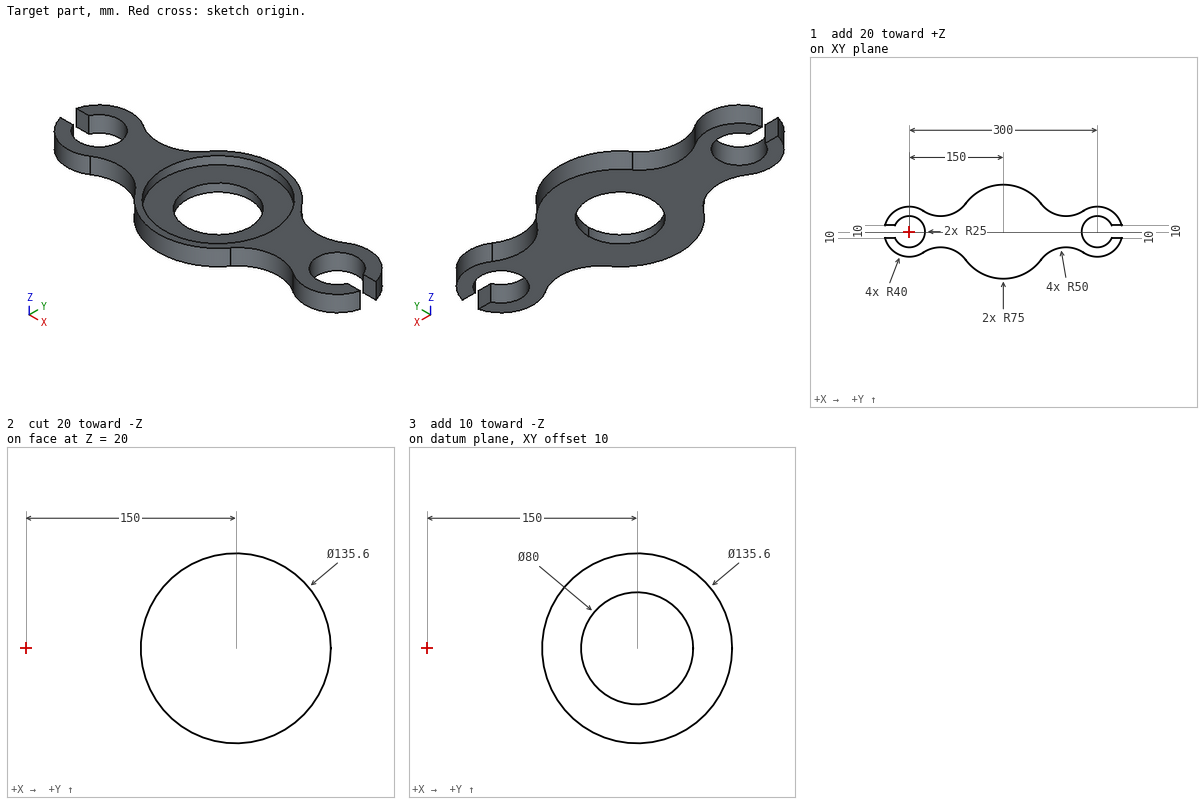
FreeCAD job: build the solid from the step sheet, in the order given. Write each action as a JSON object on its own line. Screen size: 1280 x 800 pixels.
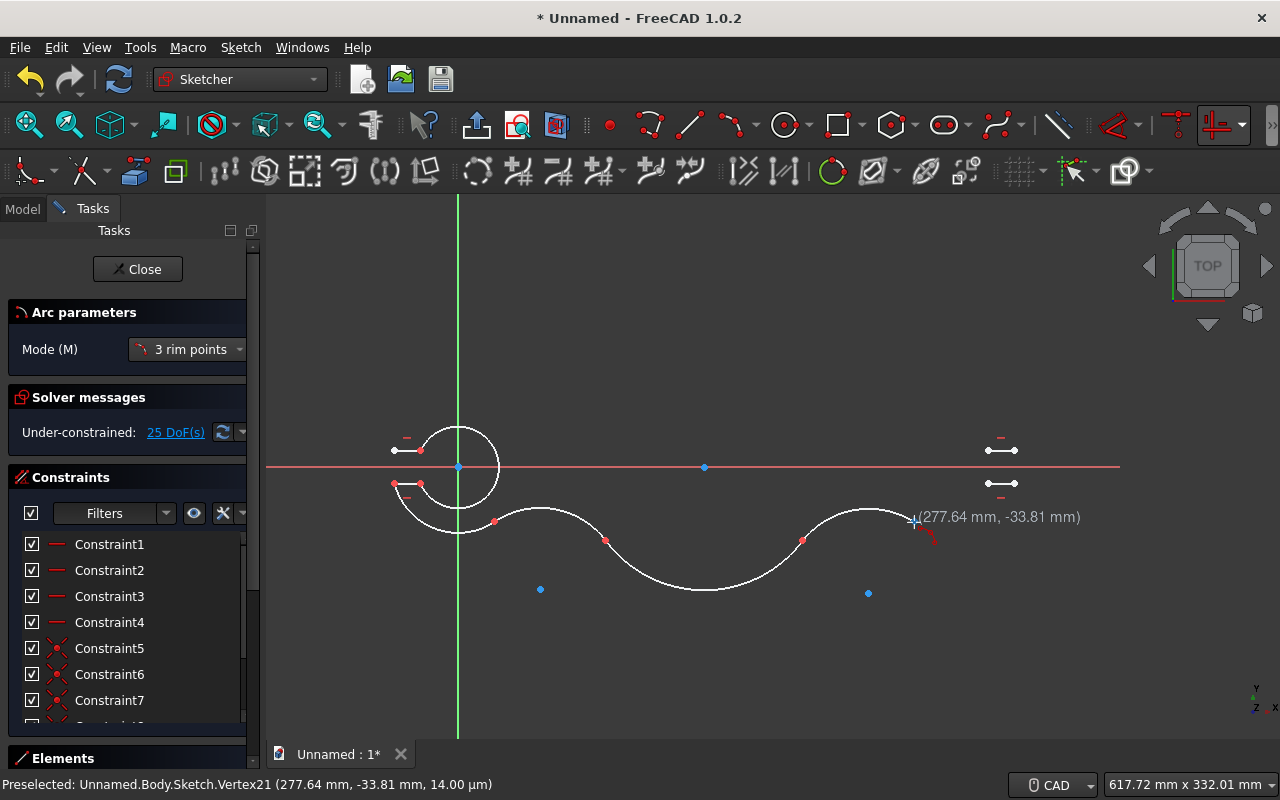
{"action": "scroll", "coordinate": [1014, 483], "scroll_direction": "up", "scroll_amount": 2}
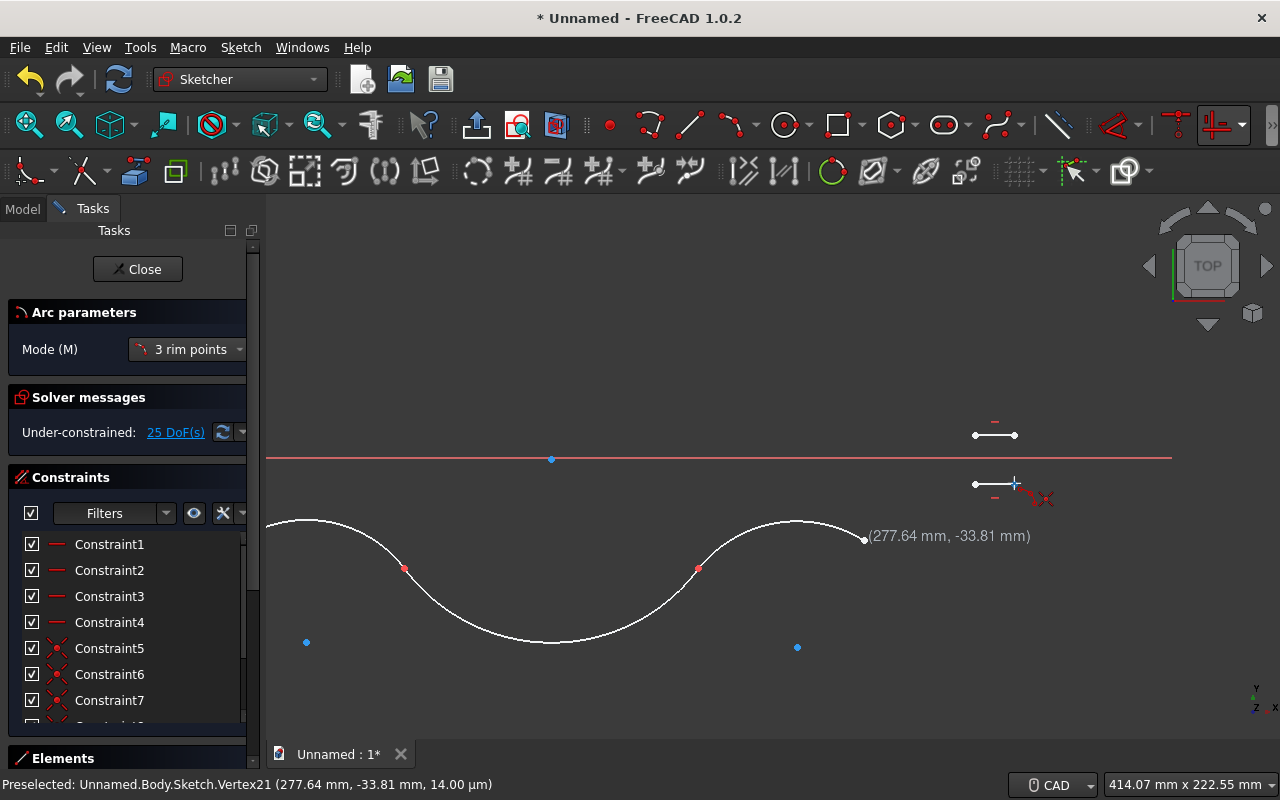
{"action": "left_click", "coordinate": [1015, 484]}
{"action": "left_click", "coordinate": [954, 550]}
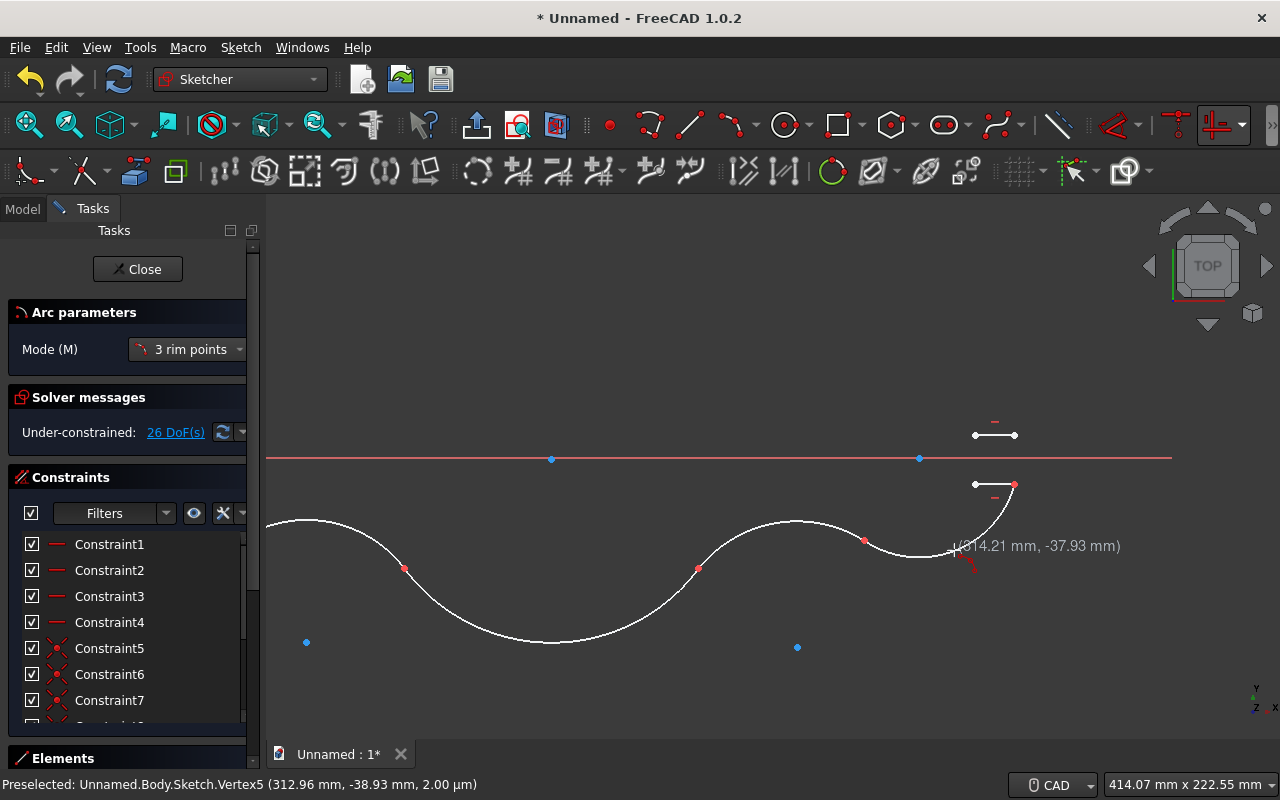
{"action": "left_click", "coordinate": [976, 484]}
{"action": "left_click", "coordinate": [976, 435]}
{"action": "left_click", "coordinate": [867, 426]}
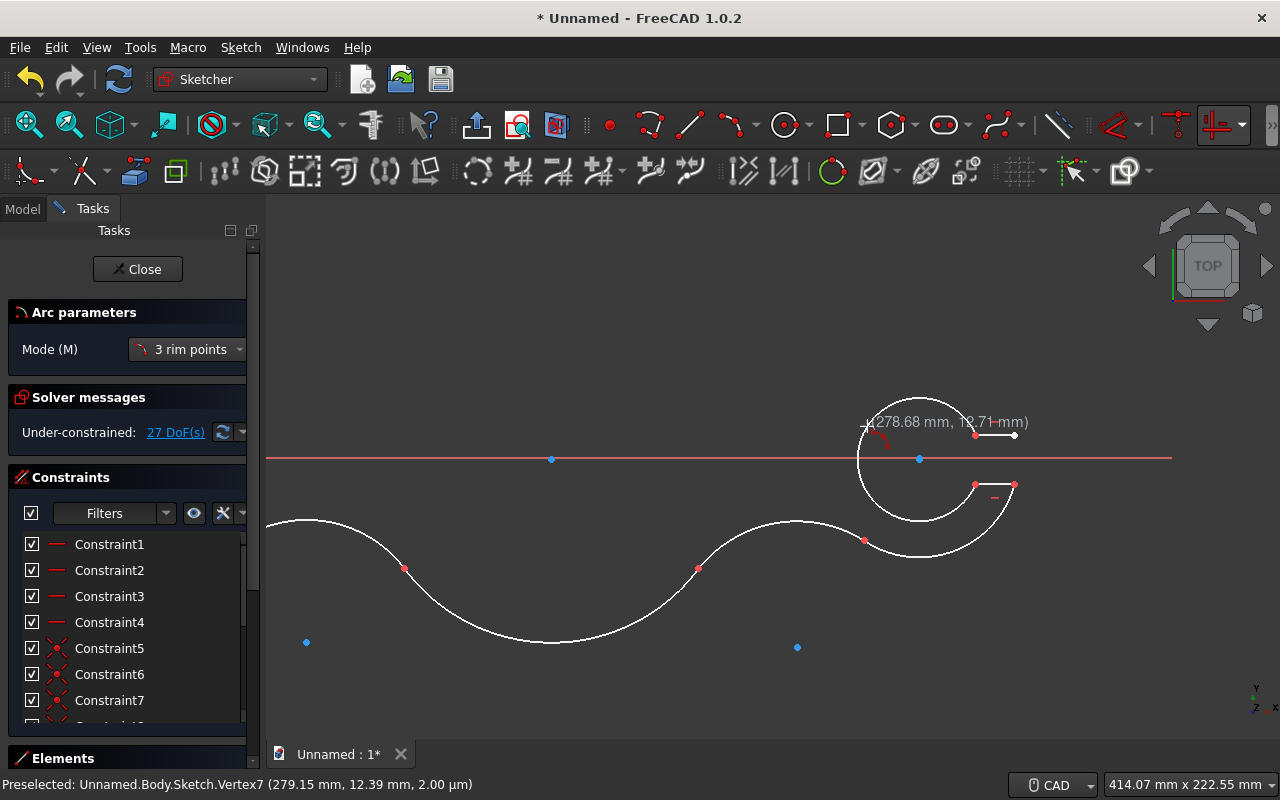
{"action": "left_click", "coordinate": [1015, 435]}
{"action": "left_click", "coordinate": [865, 377]}
{"action": "left_click", "coordinate": [954, 367]}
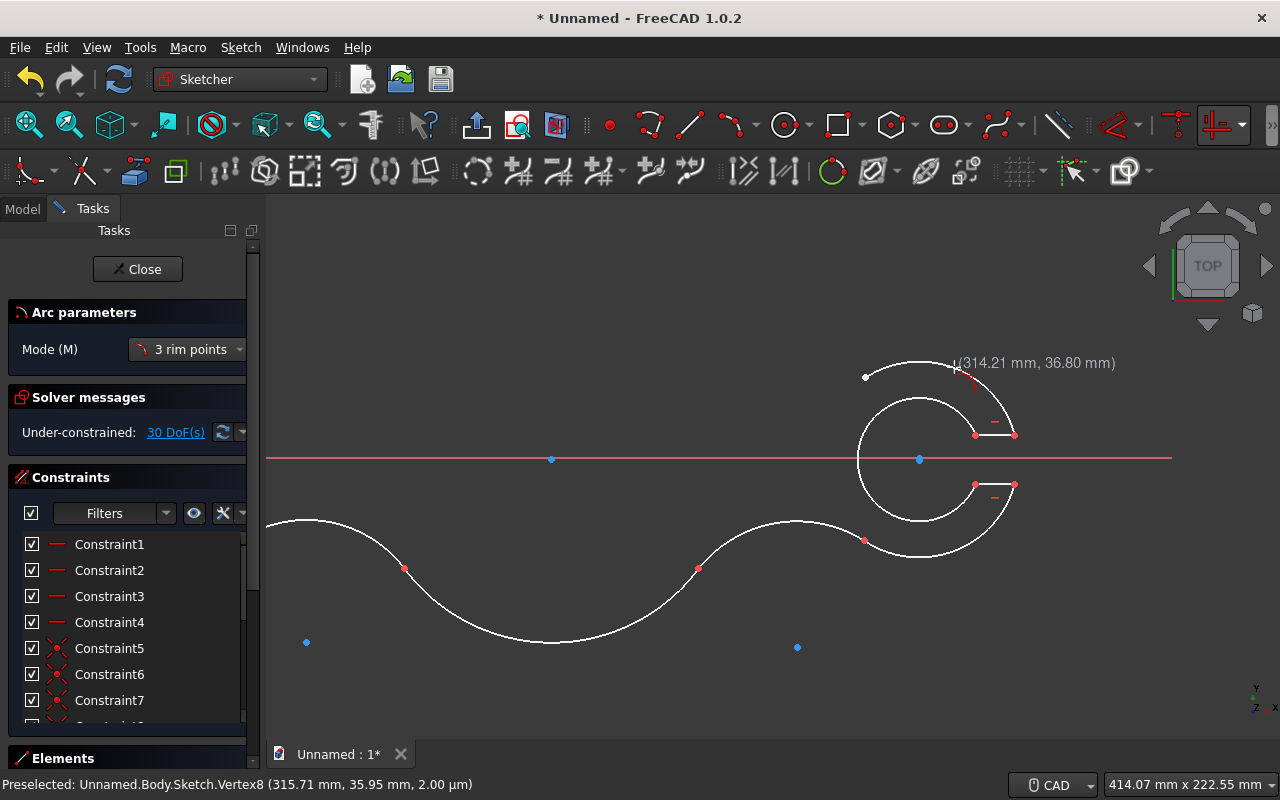
{"action": "left_click", "coordinate": [865, 378]}
{"action": "left_click", "coordinate": [699, 348]}
{"action": "left_click", "coordinate": [776, 395]}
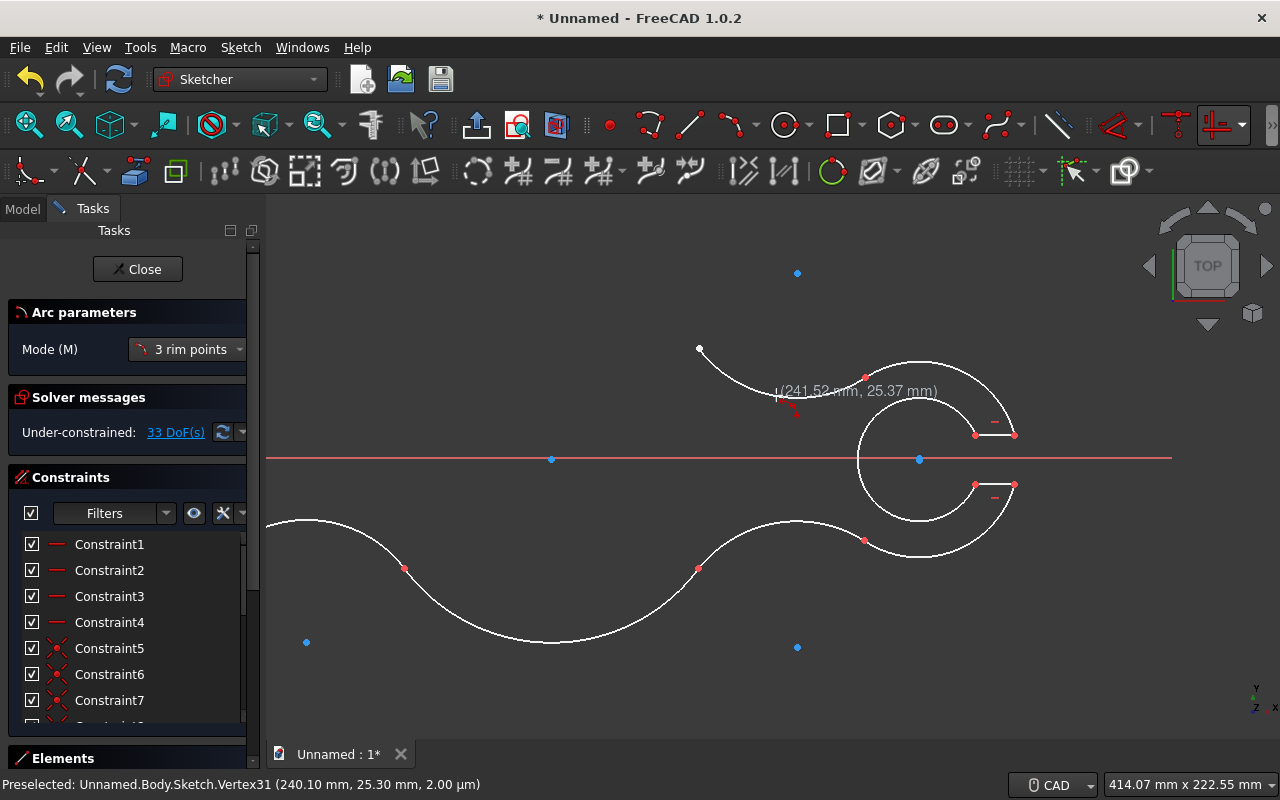
{"action": "left_click", "coordinate": [699, 349]}
{"action": "left_click", "coordinate": [405, 348]}
{"action": "left_click", "coordinate": [552, 274]}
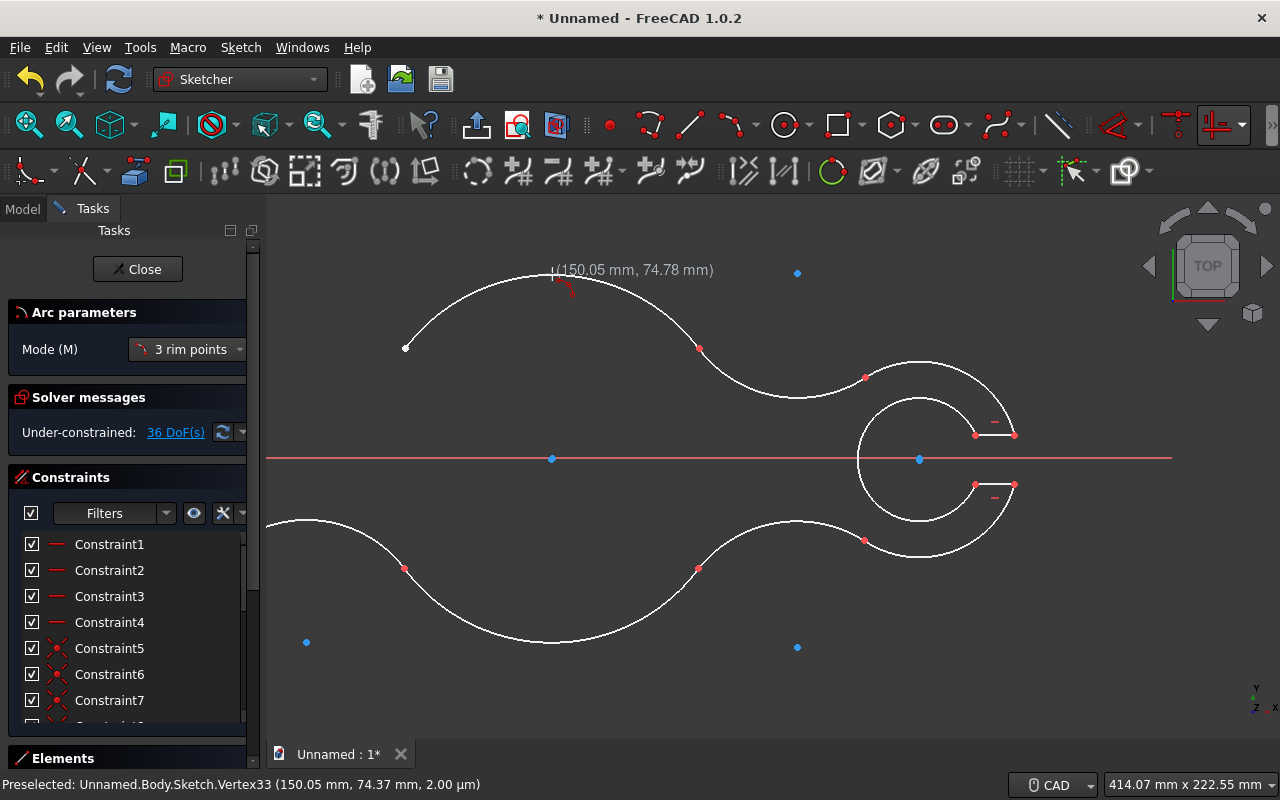
{"action": "left_click", "coordinate": [405, 349]}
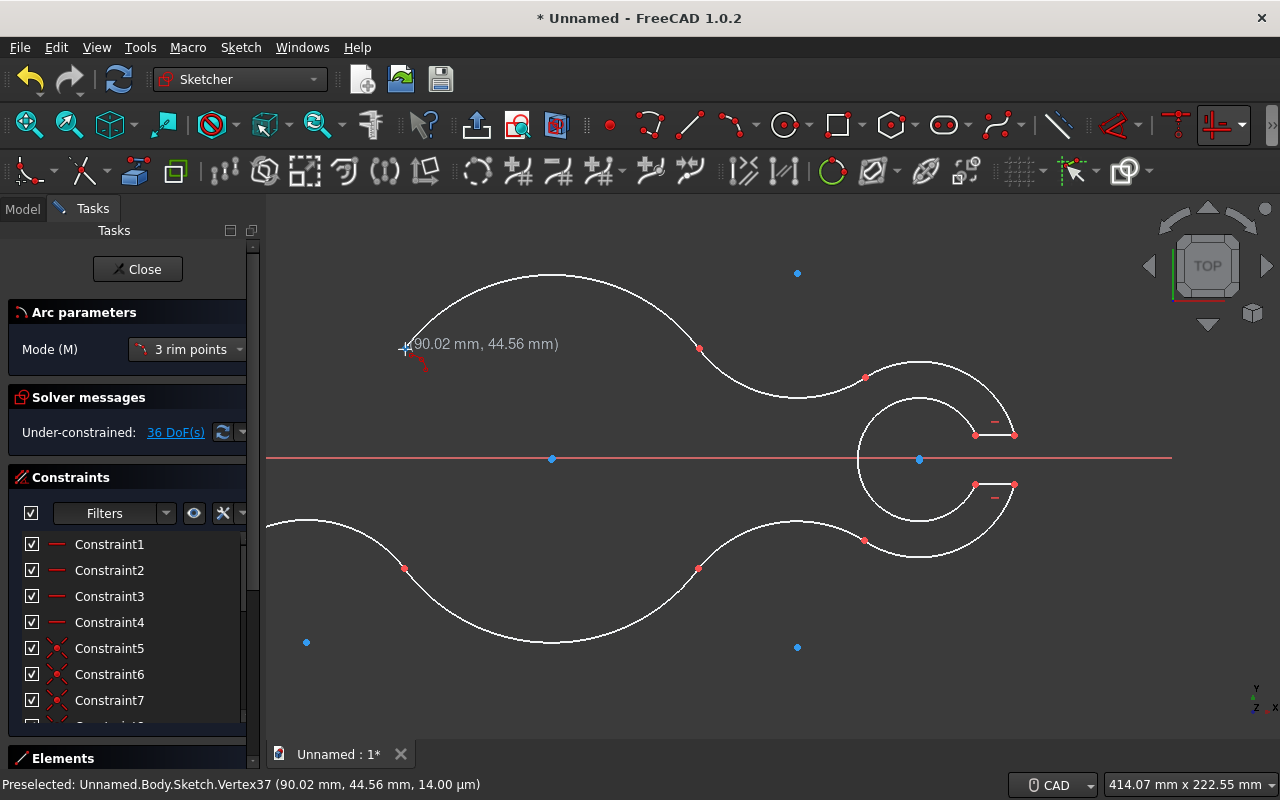
{"action": "scroll", "coordinate": [1015, 484], "scroll_direction": "down", "scroll_amount": 2}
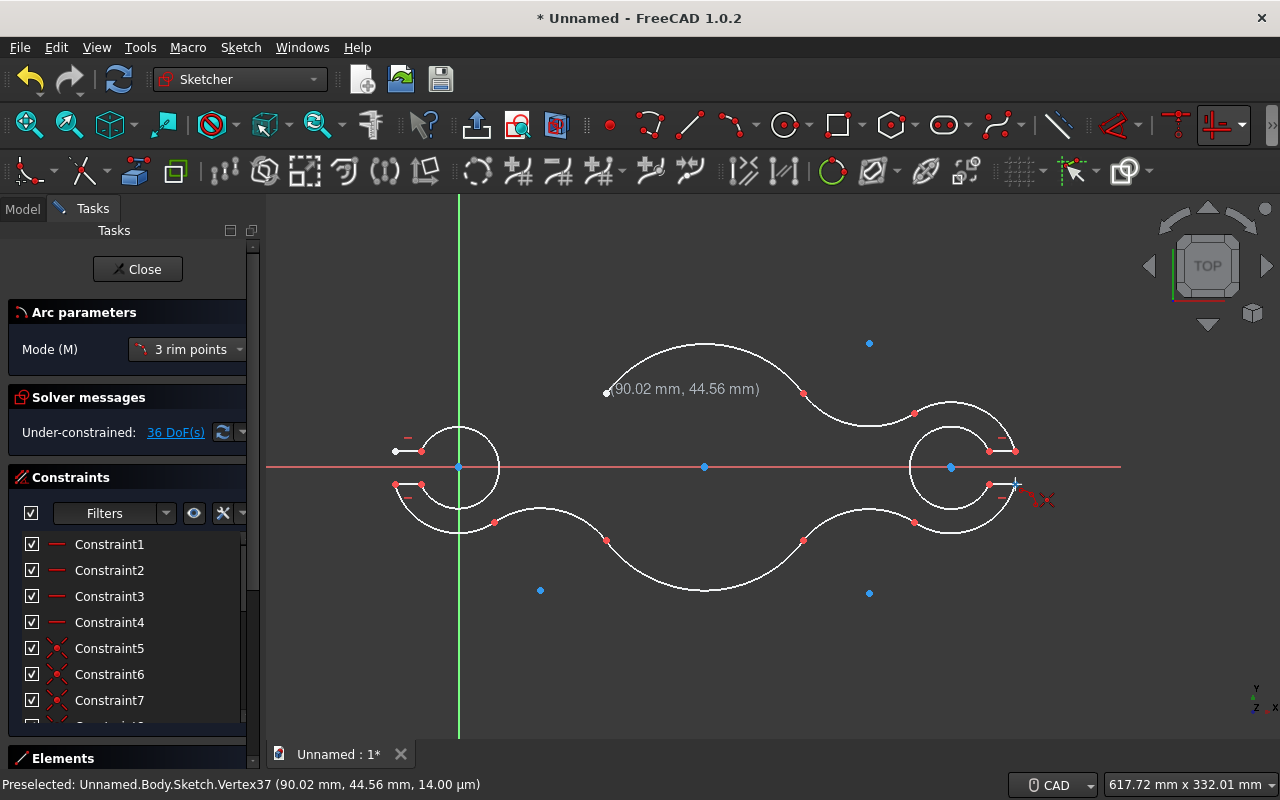
{"action": "left_click", "coordinate": [495, 412]}
{"action": "left_click", "coordinate": [554, 425]}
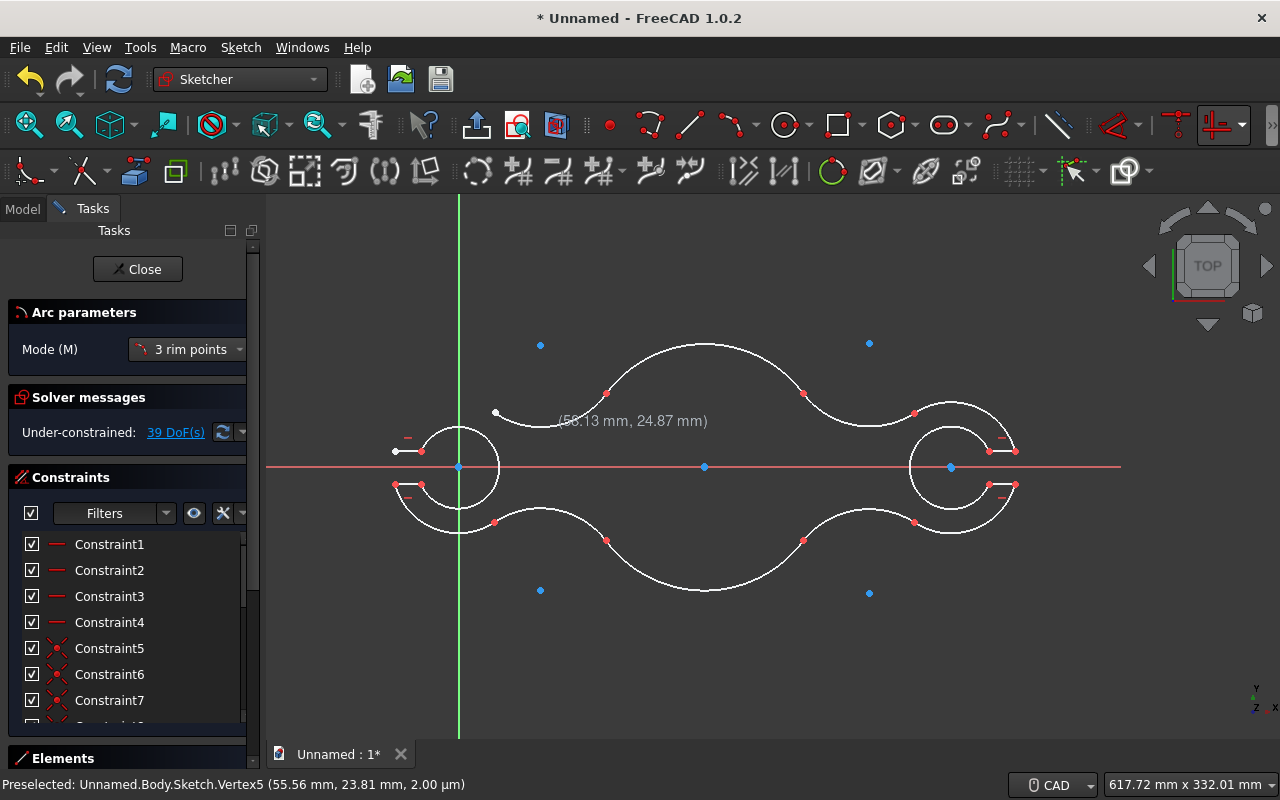
{"action": "left_click", "coordinate": [495, 413]}